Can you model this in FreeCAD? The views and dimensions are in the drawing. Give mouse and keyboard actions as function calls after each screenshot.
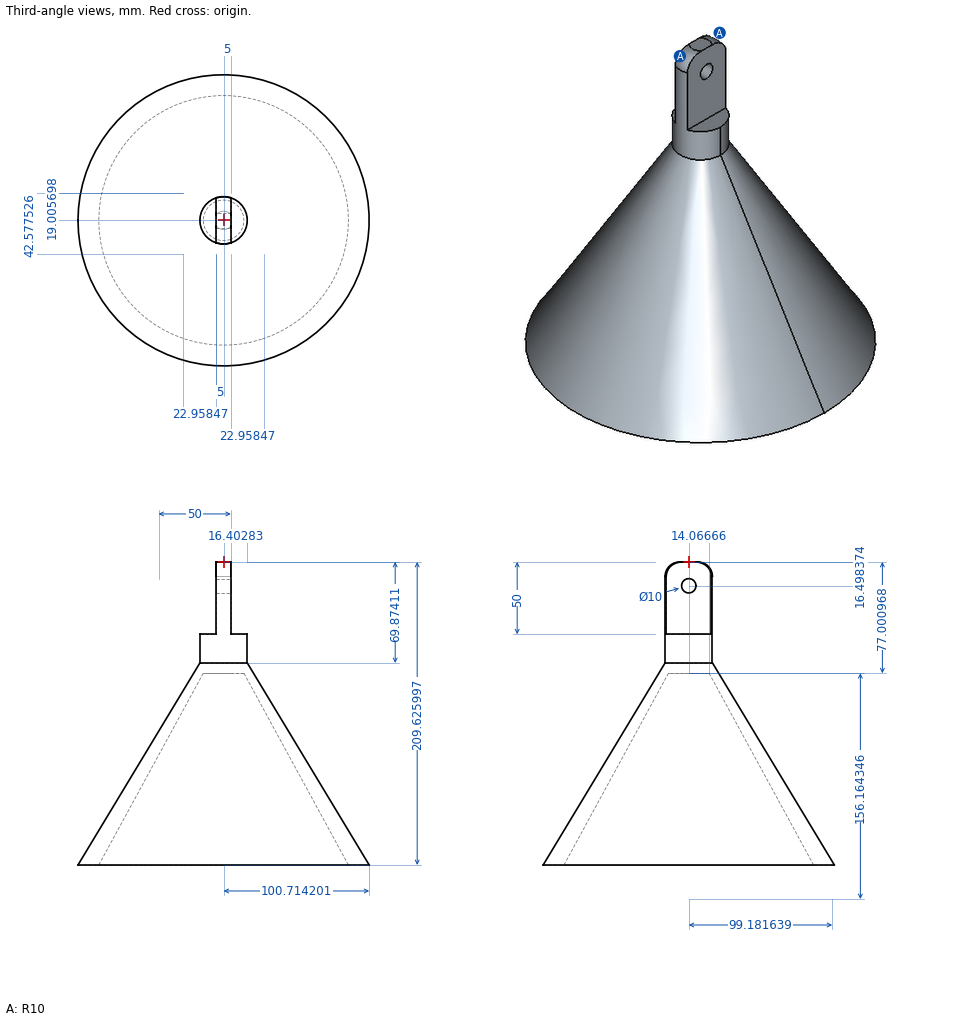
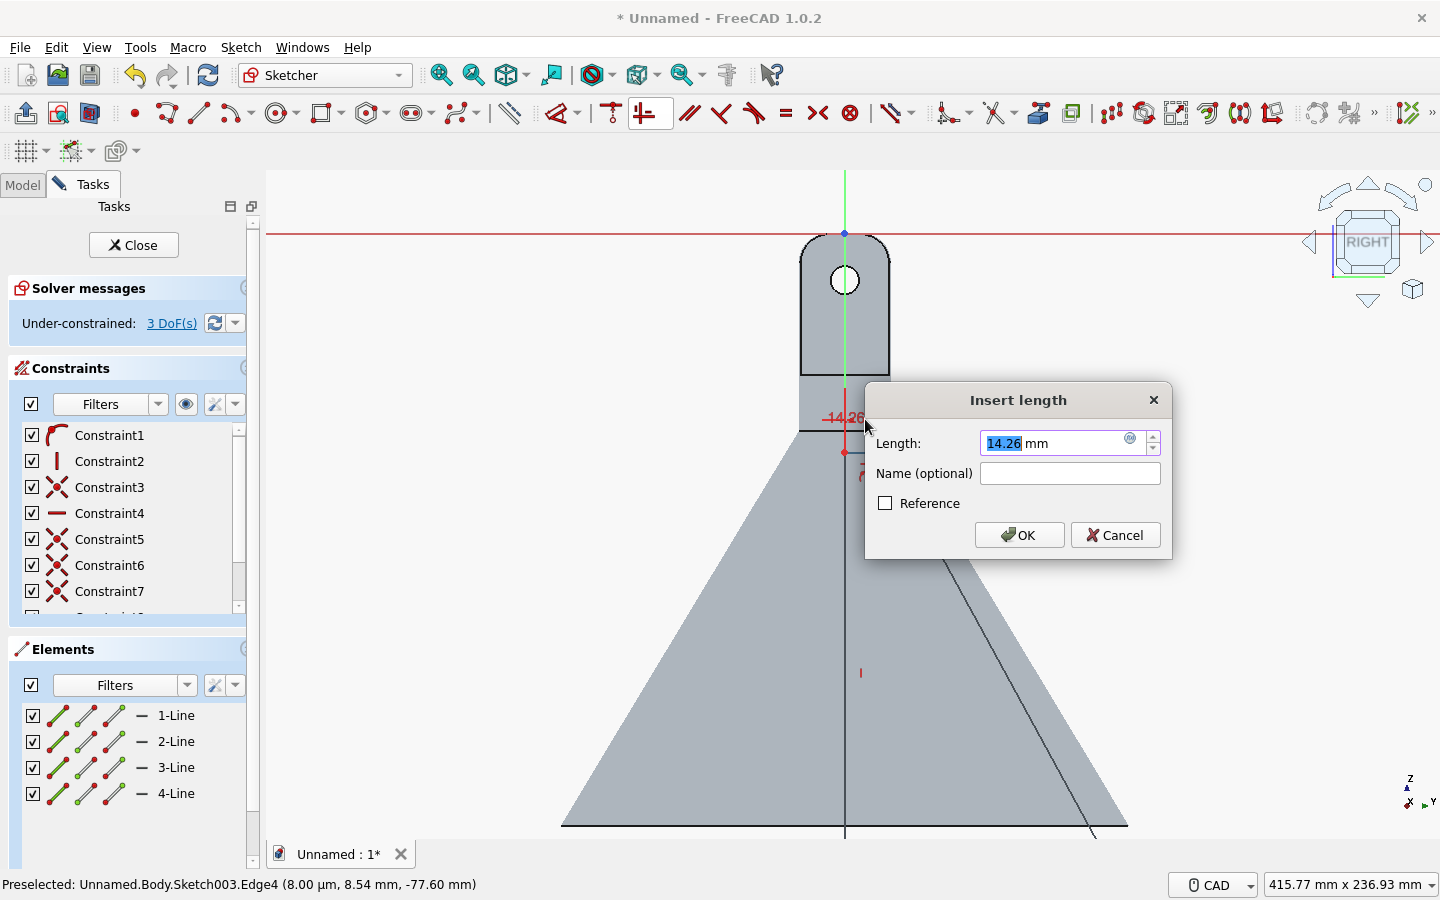
text(14.06666)
key(Return)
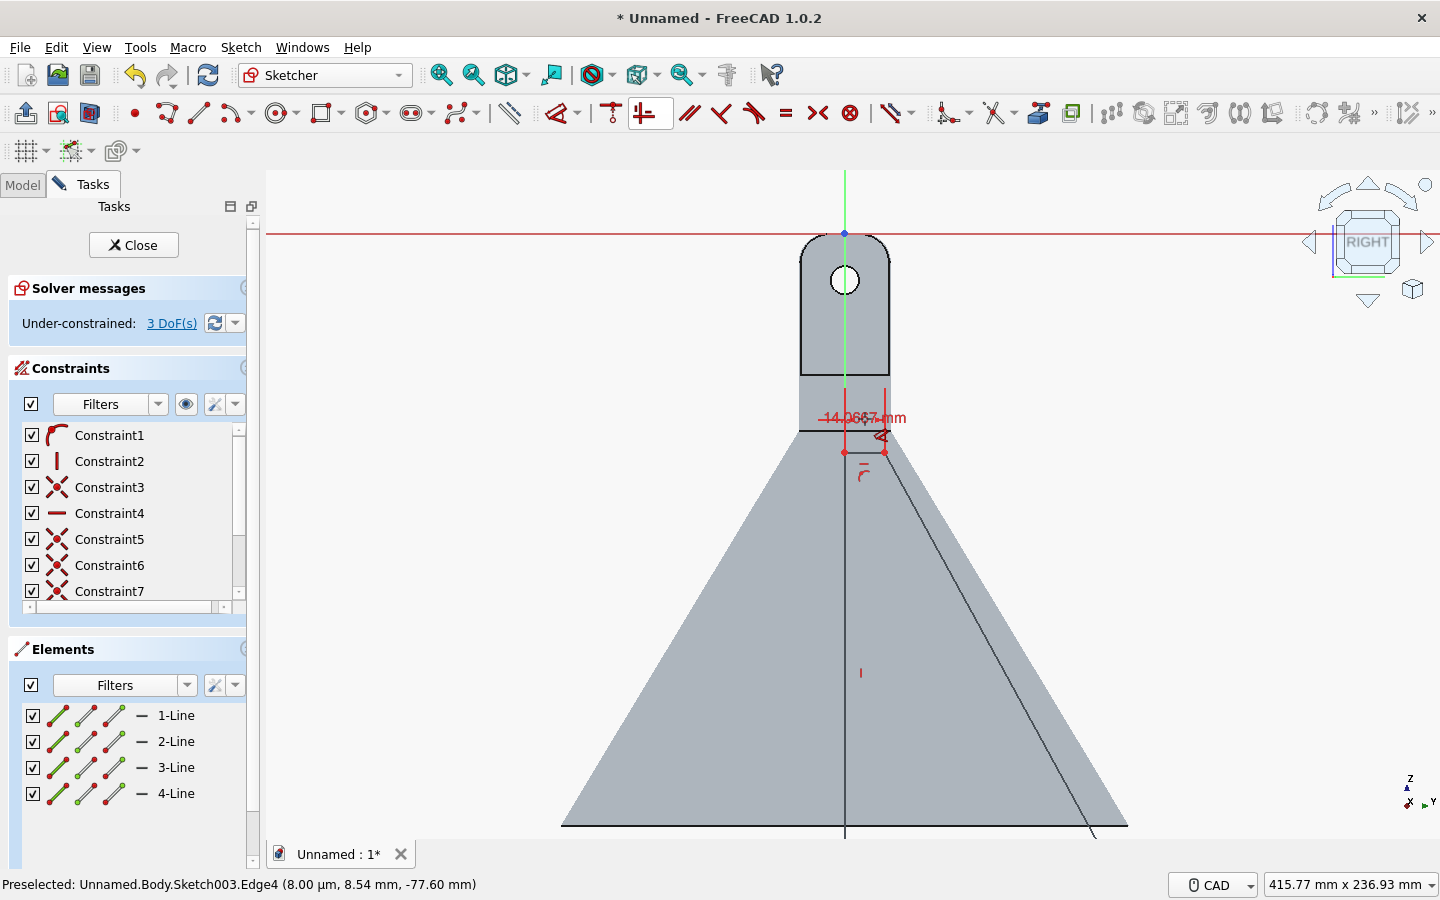
scroll(377, 386, down, 2)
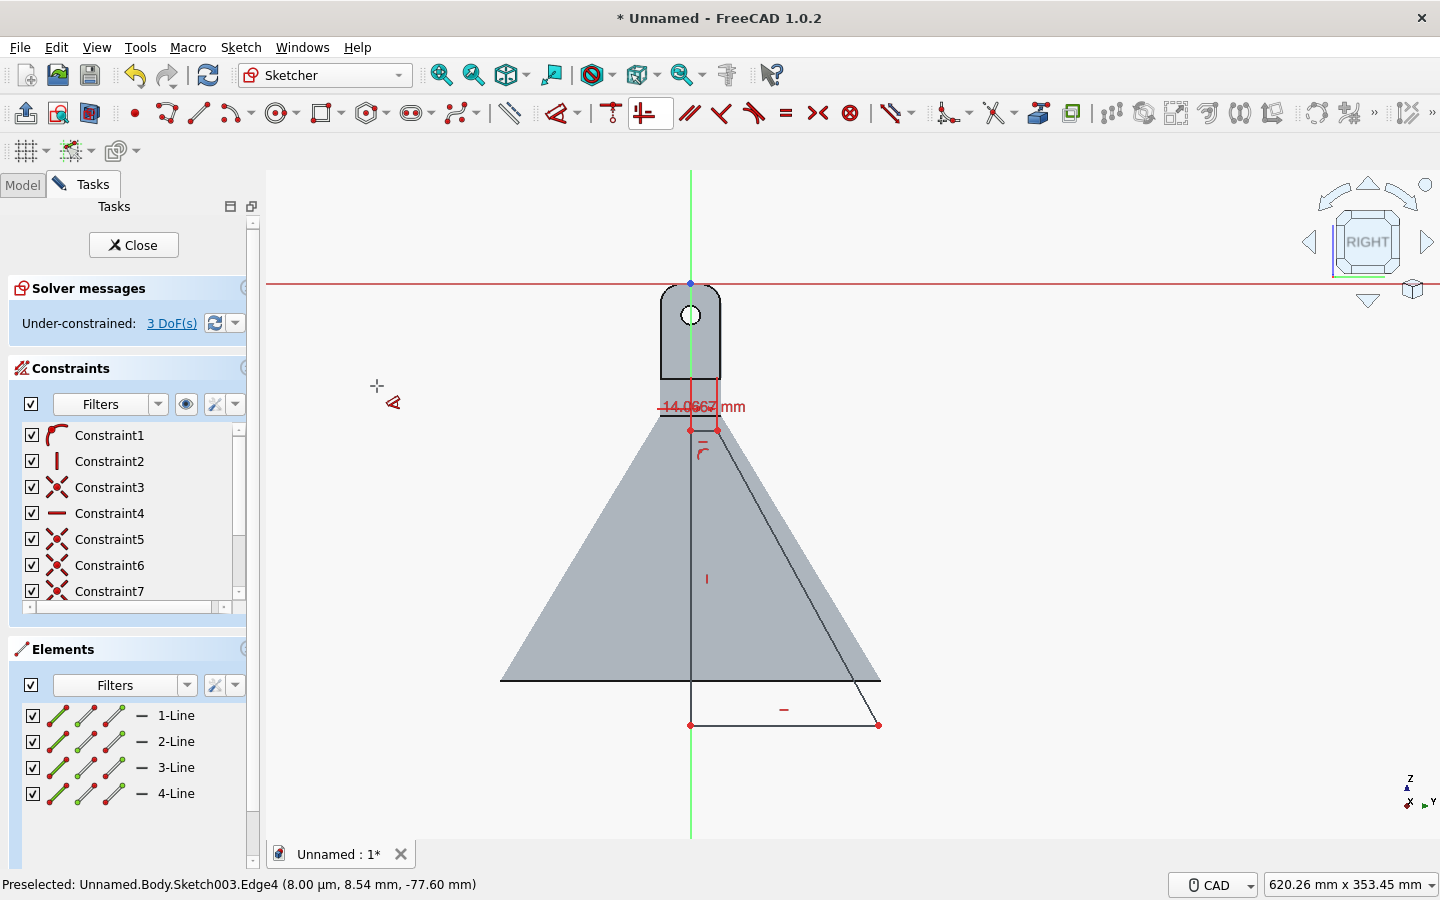
click(747, 726)
click(785, 760)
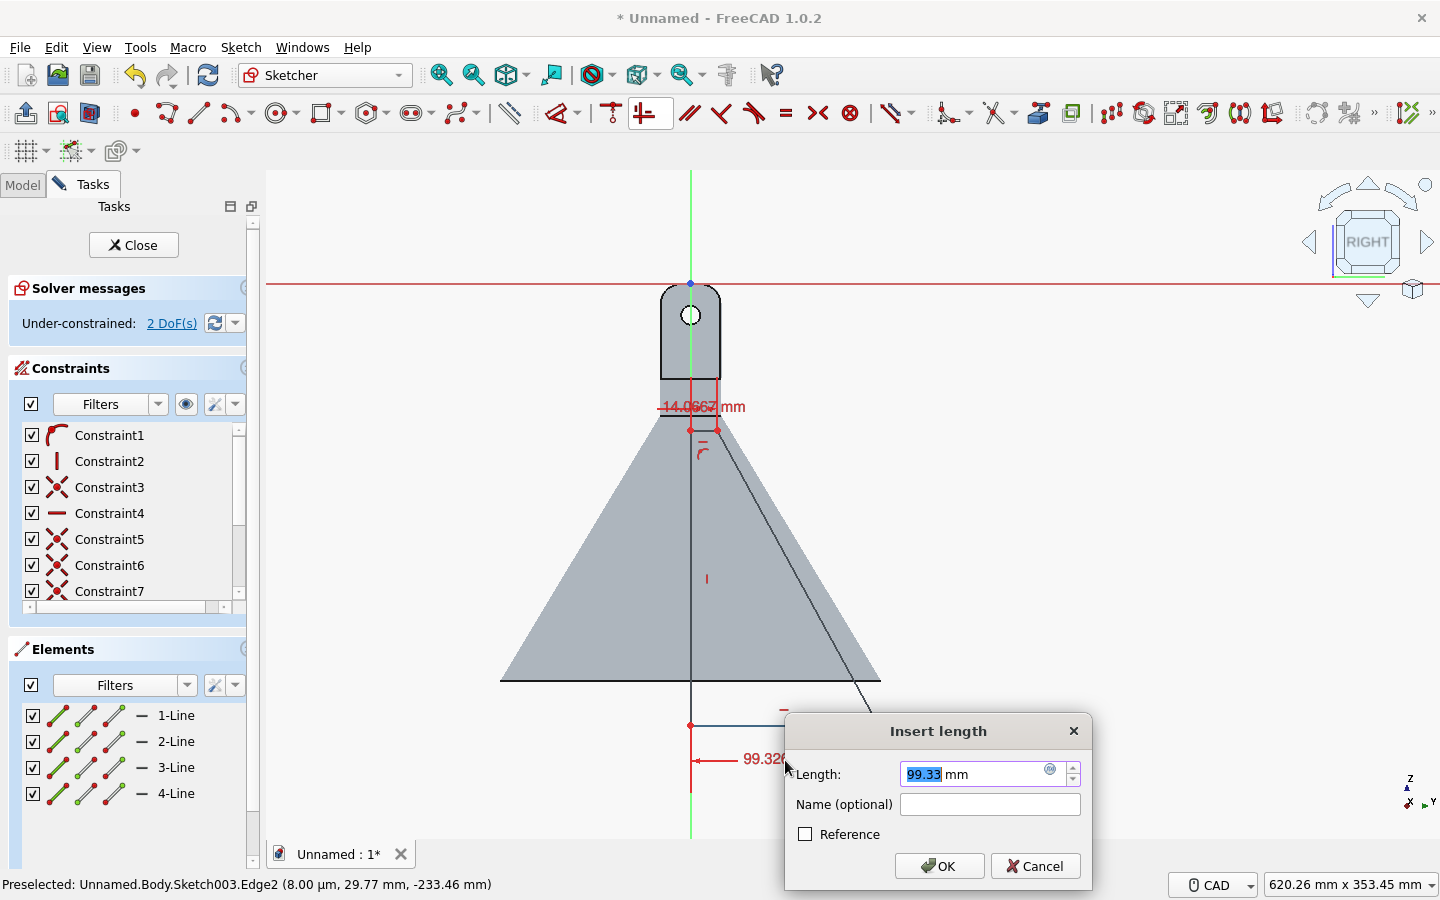
text(99.181639)
key(Return)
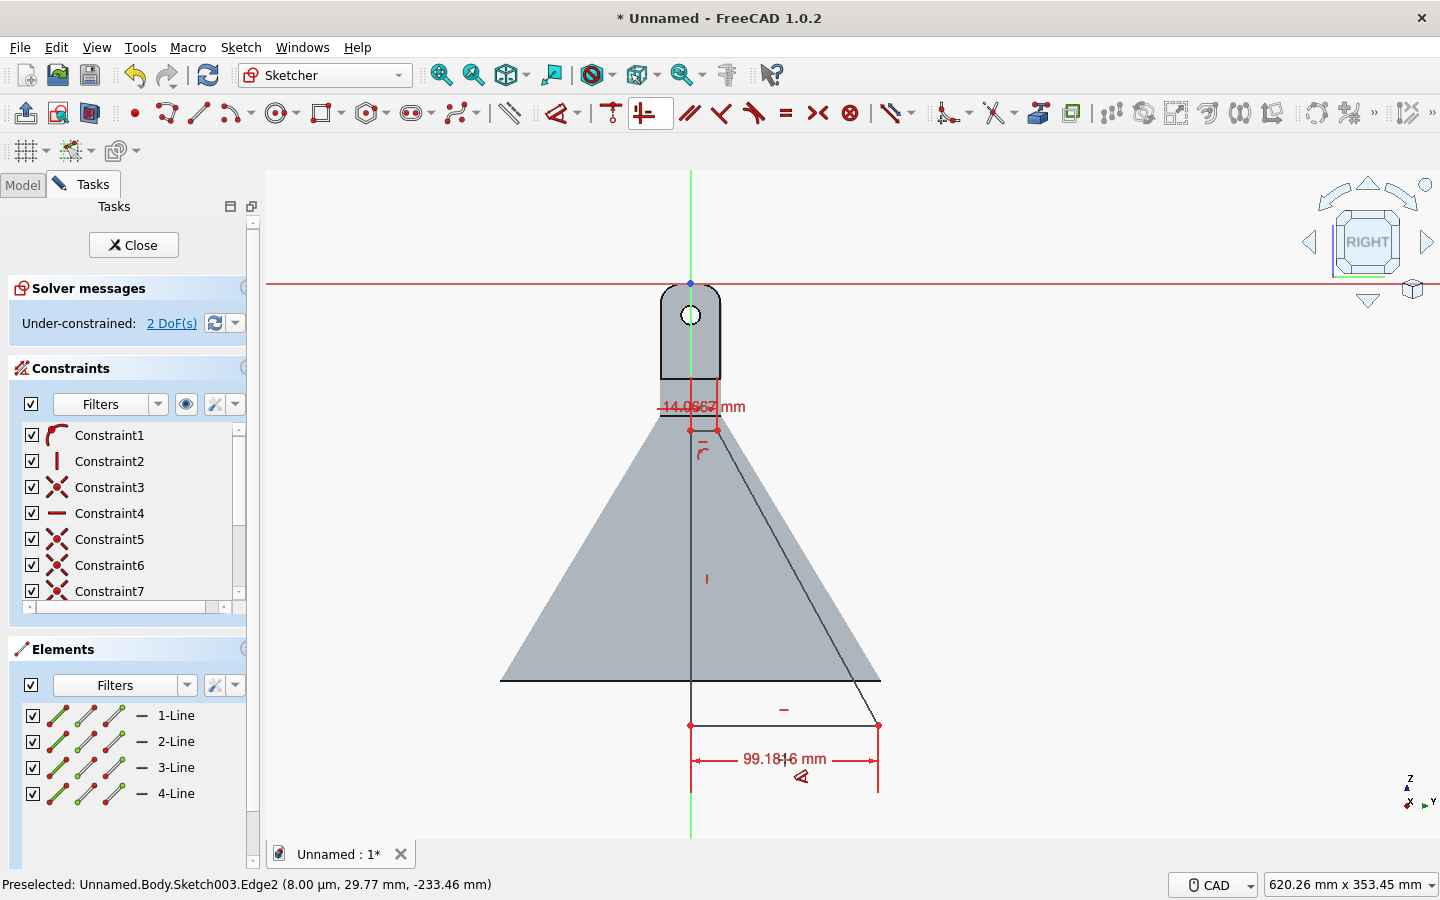
click(691, 519)
click(657, 578)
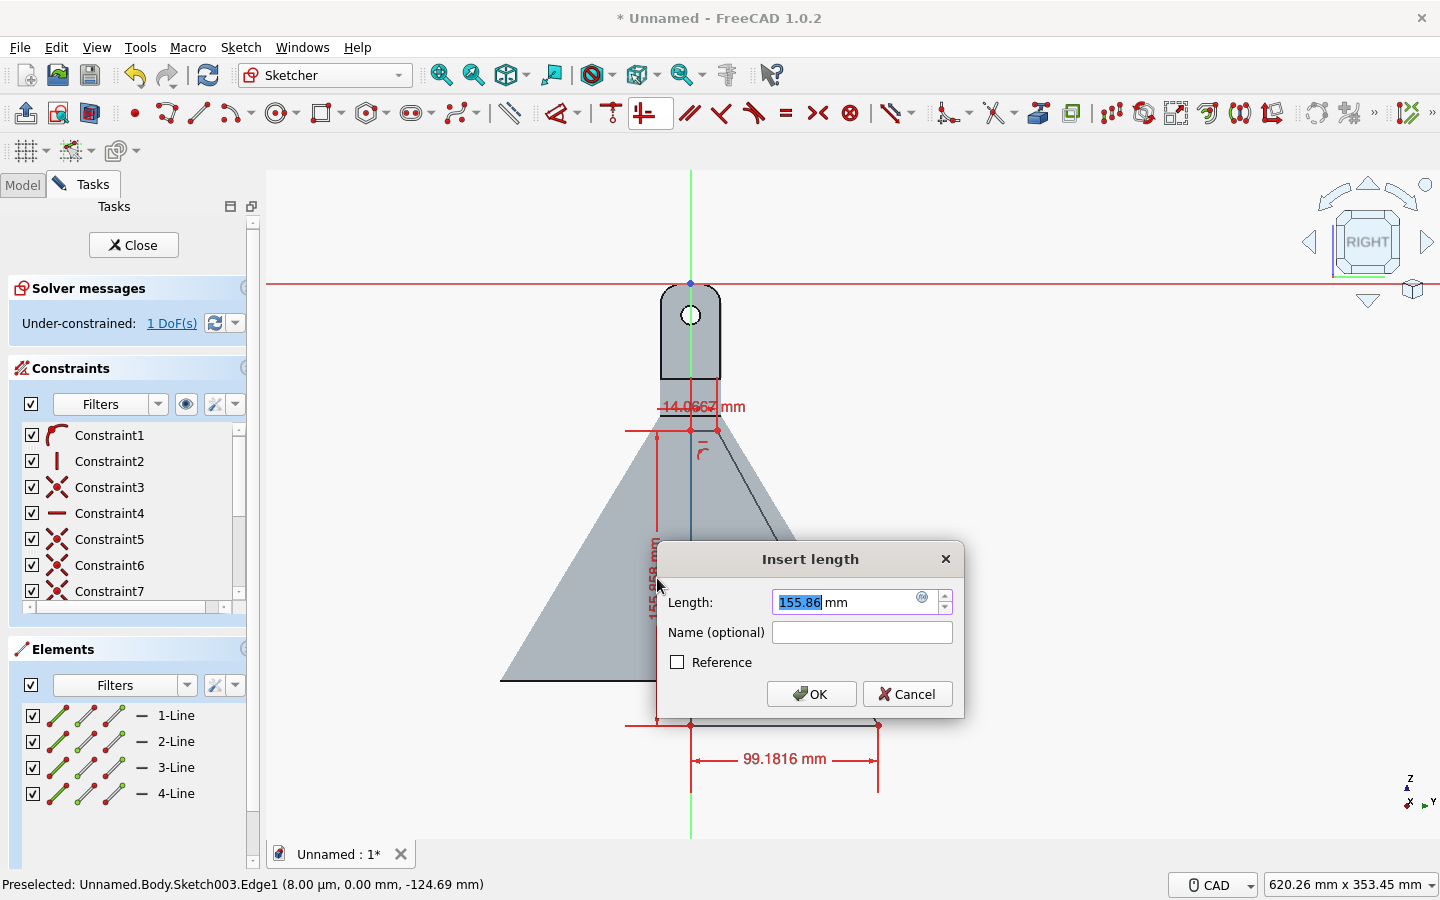
text(156.164346)
key(Return)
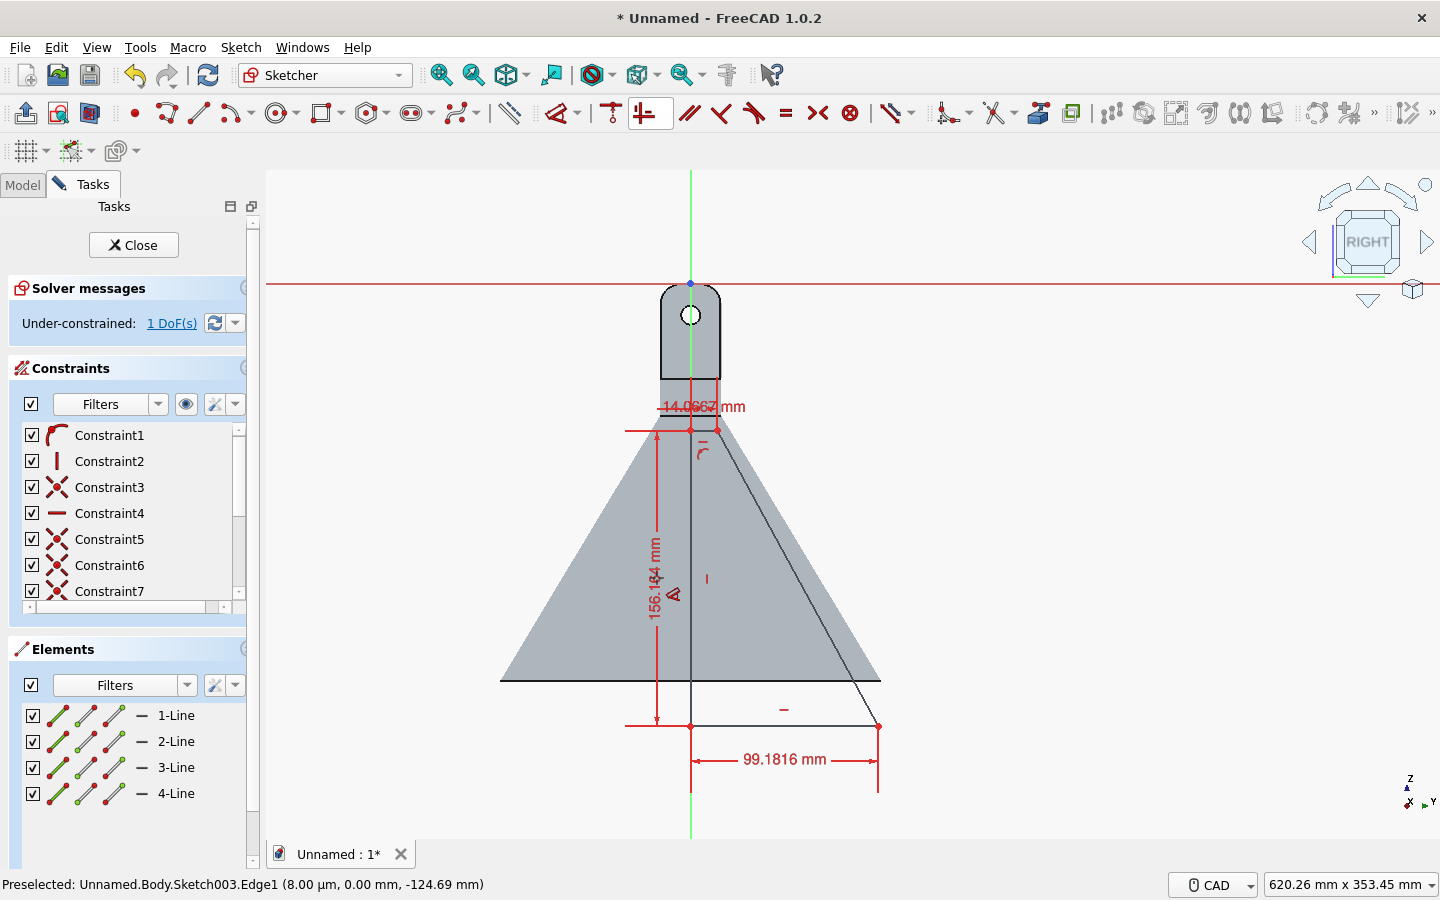
click(691, 431)
click(657, 357)